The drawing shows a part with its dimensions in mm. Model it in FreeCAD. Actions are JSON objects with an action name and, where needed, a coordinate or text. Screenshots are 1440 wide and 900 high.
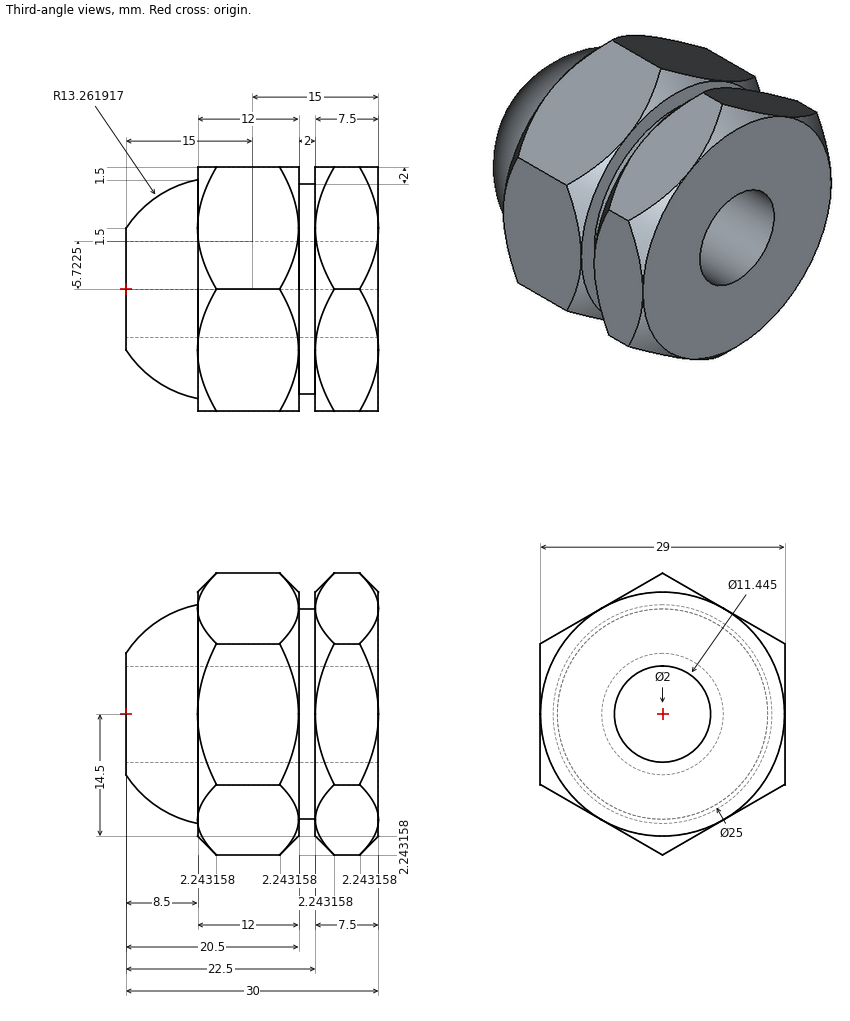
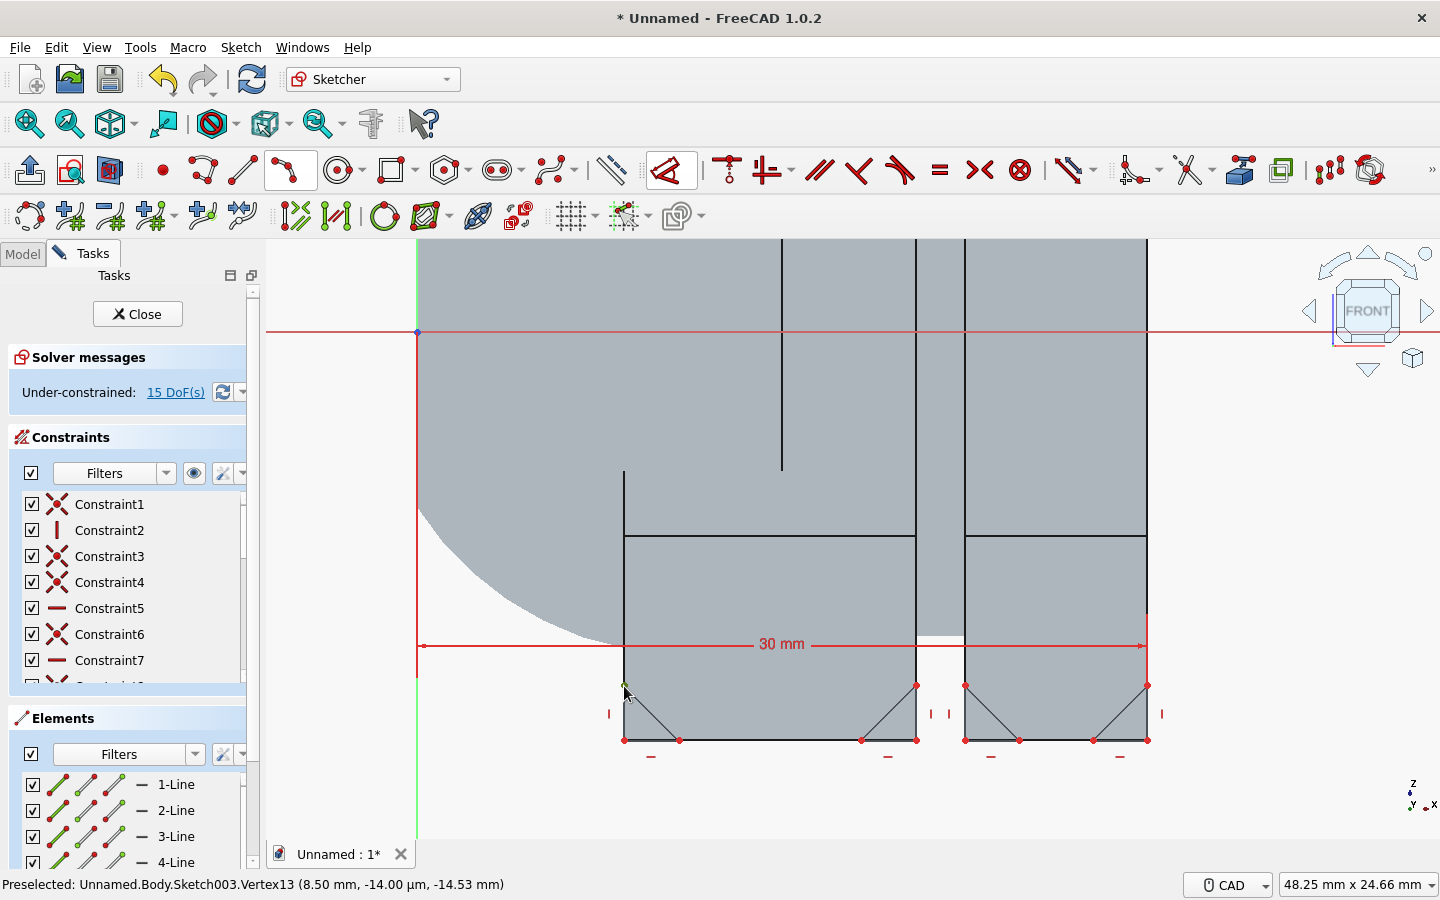
{"action": "left_click", "coordinate": [692, 170]}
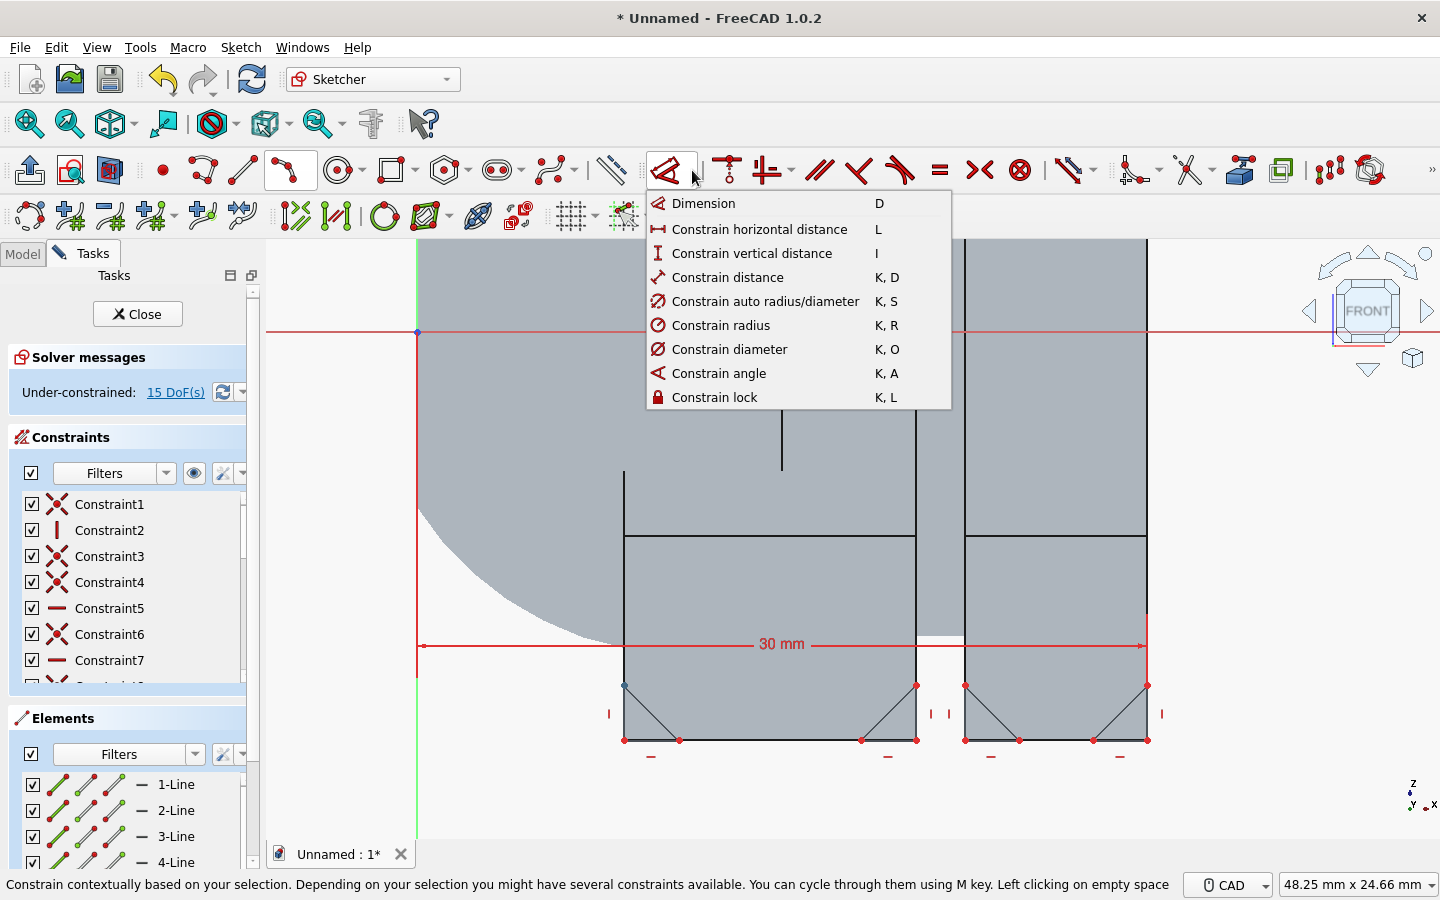
{"action": "left_click", "coordinate": [799, 229]}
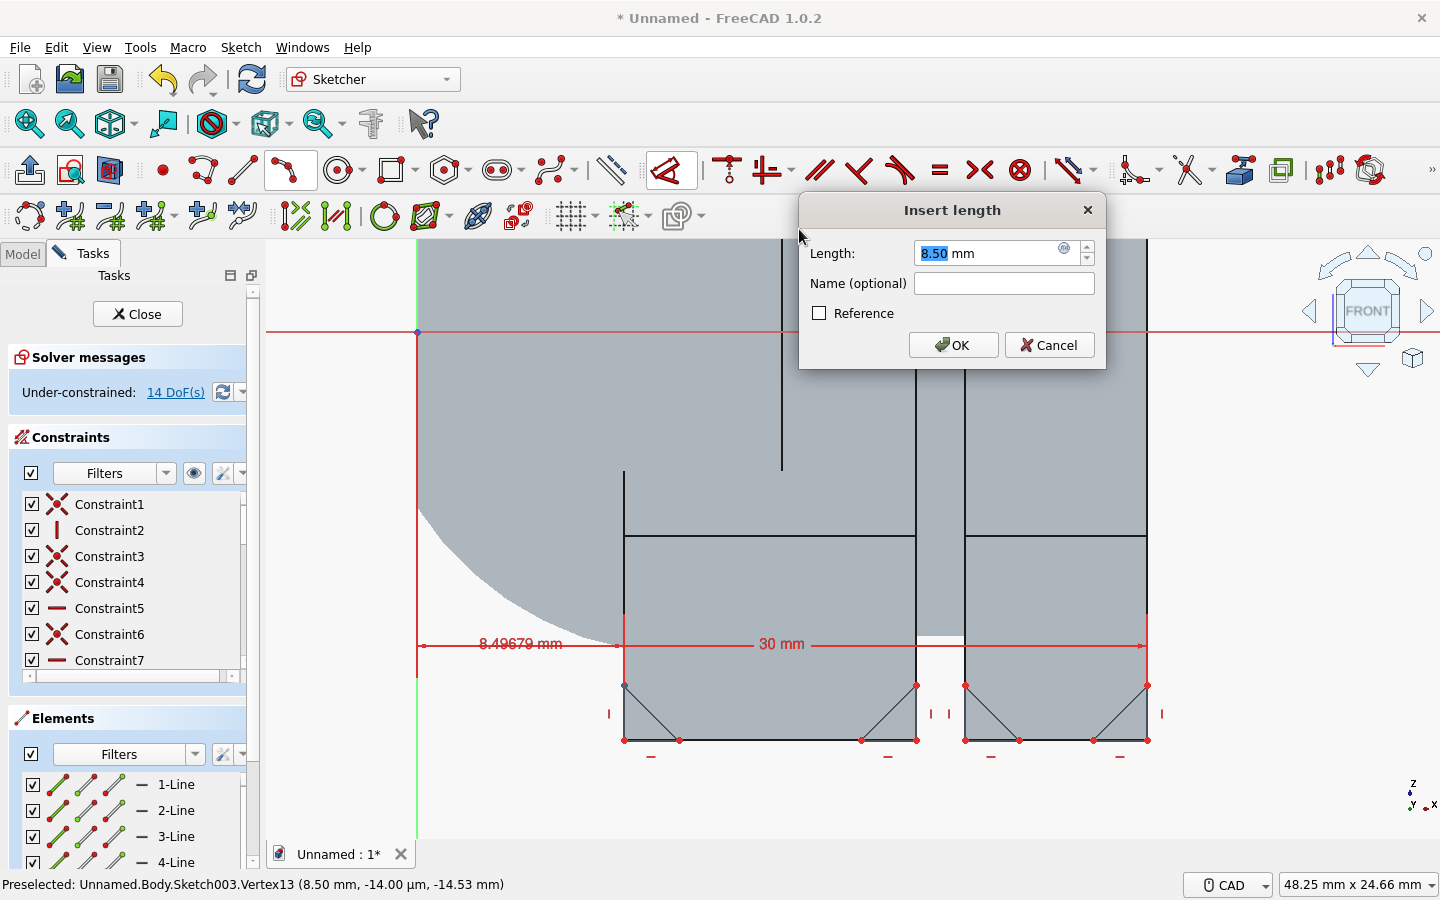
{"action": "type", "text": "8.5"}
{"action": "key", "text": "Return"}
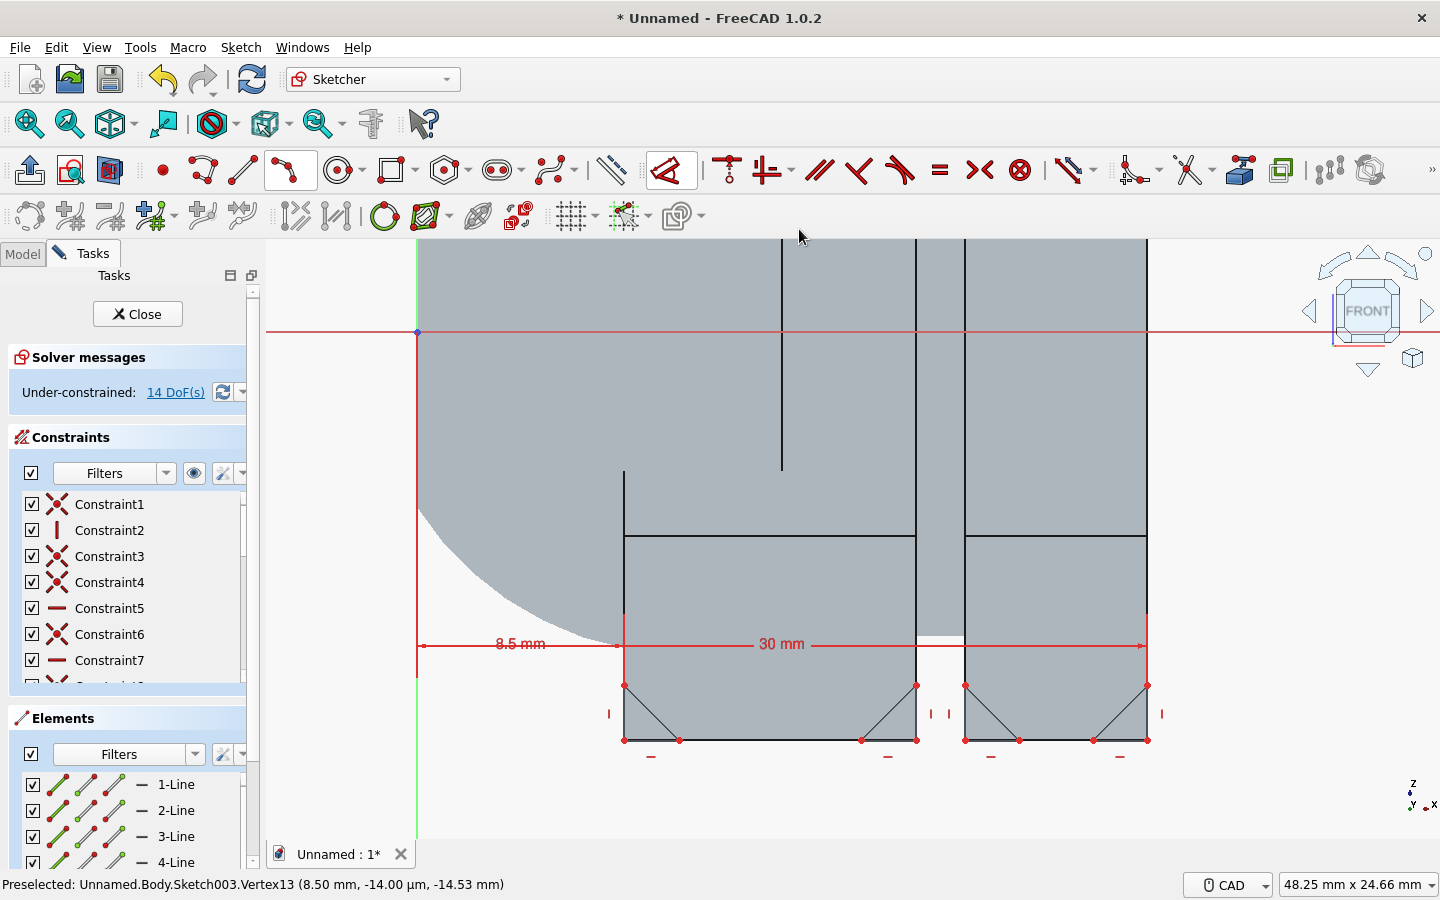
{"action": "left_click", "coordinate": [916, 686]}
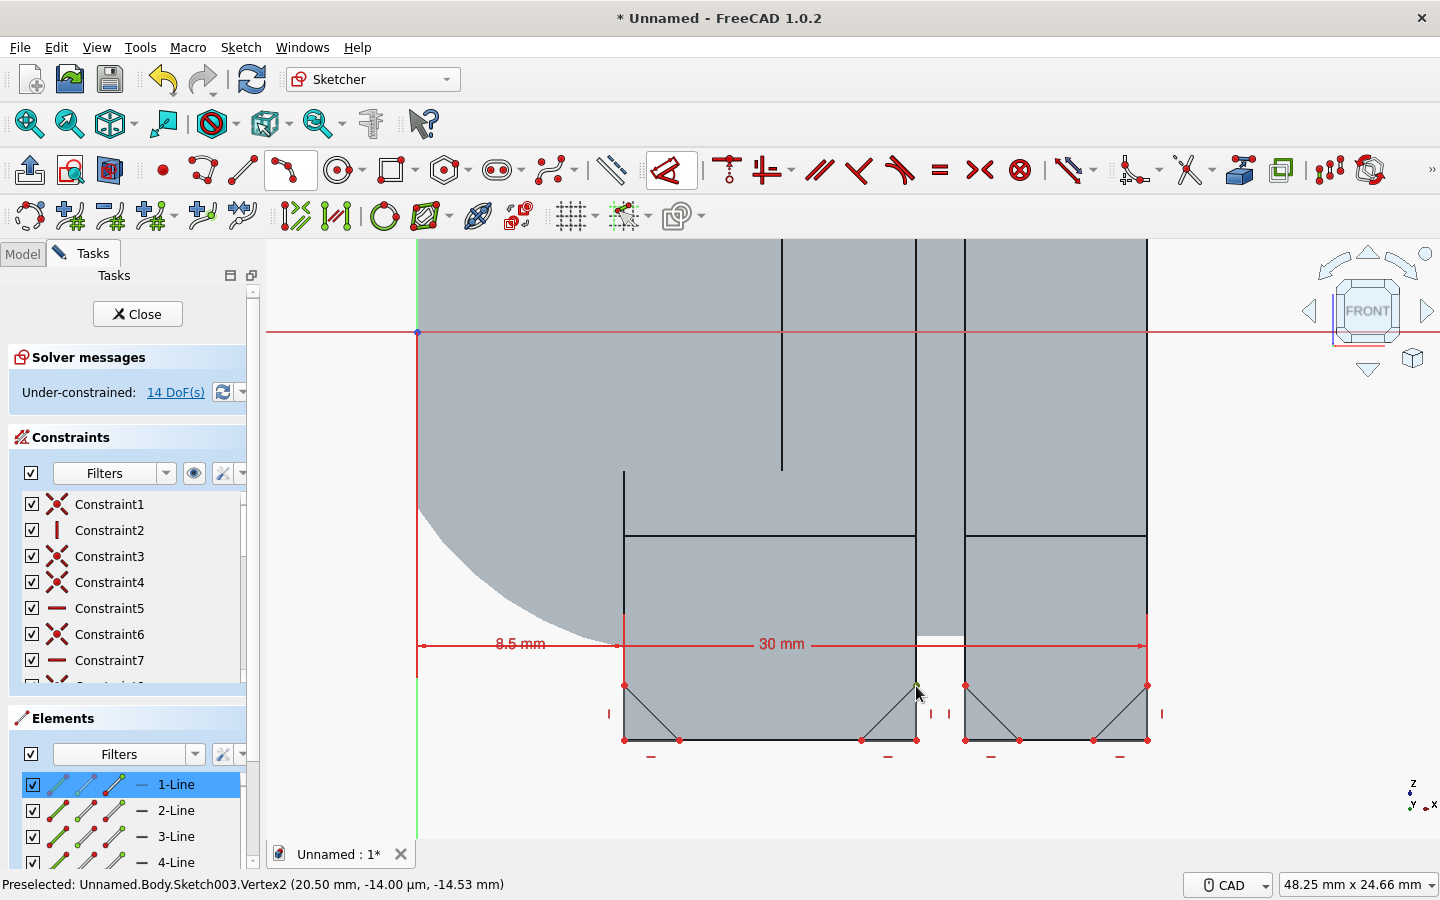
{"action": "left_click", "coordinate": [692, 170]}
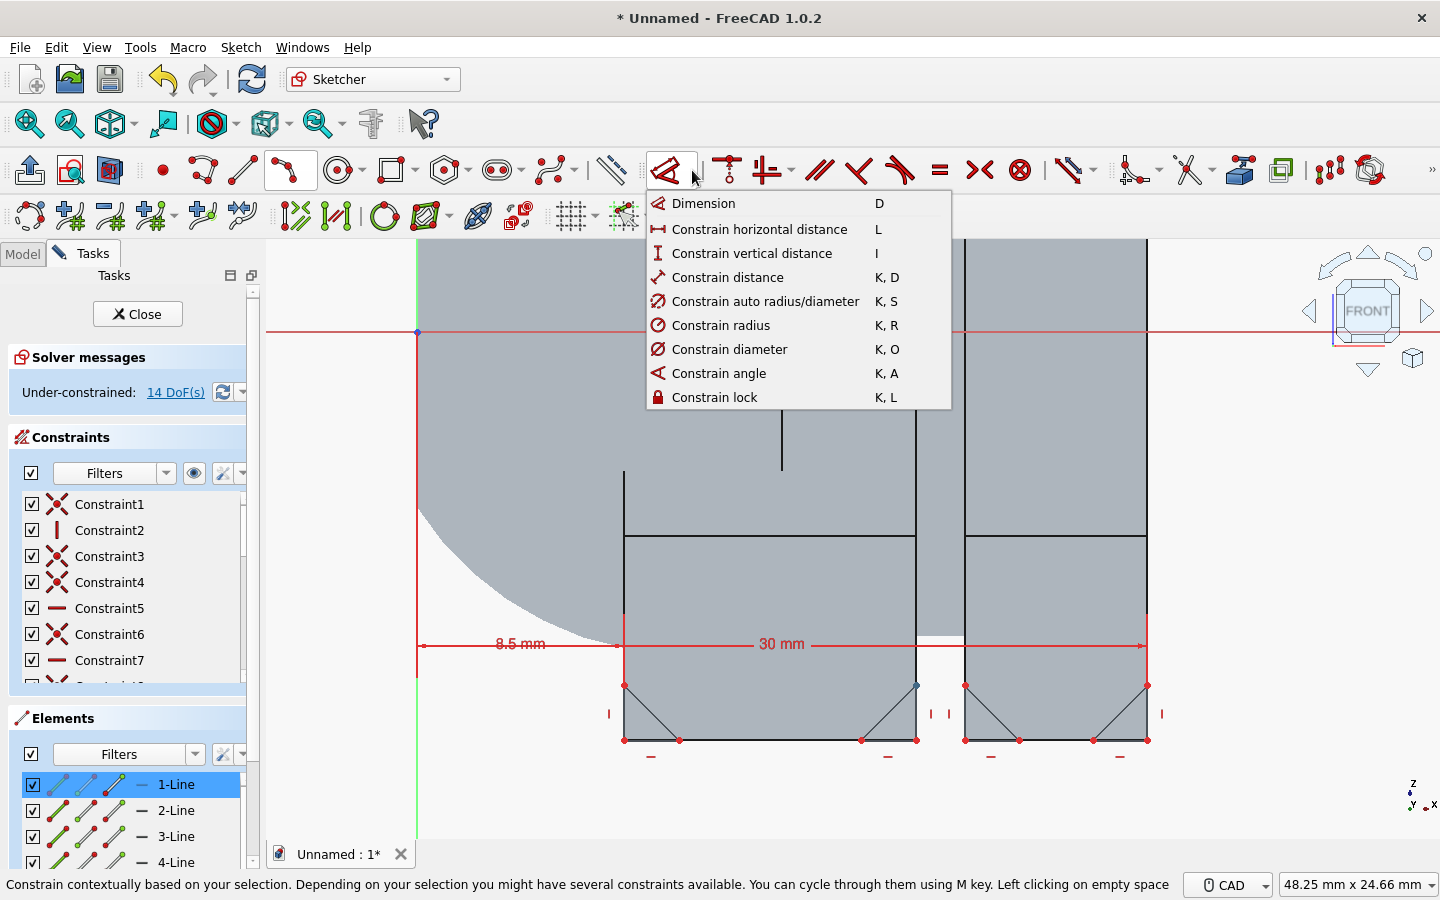
{"action": "left_click", "coordinate": [799, 229]}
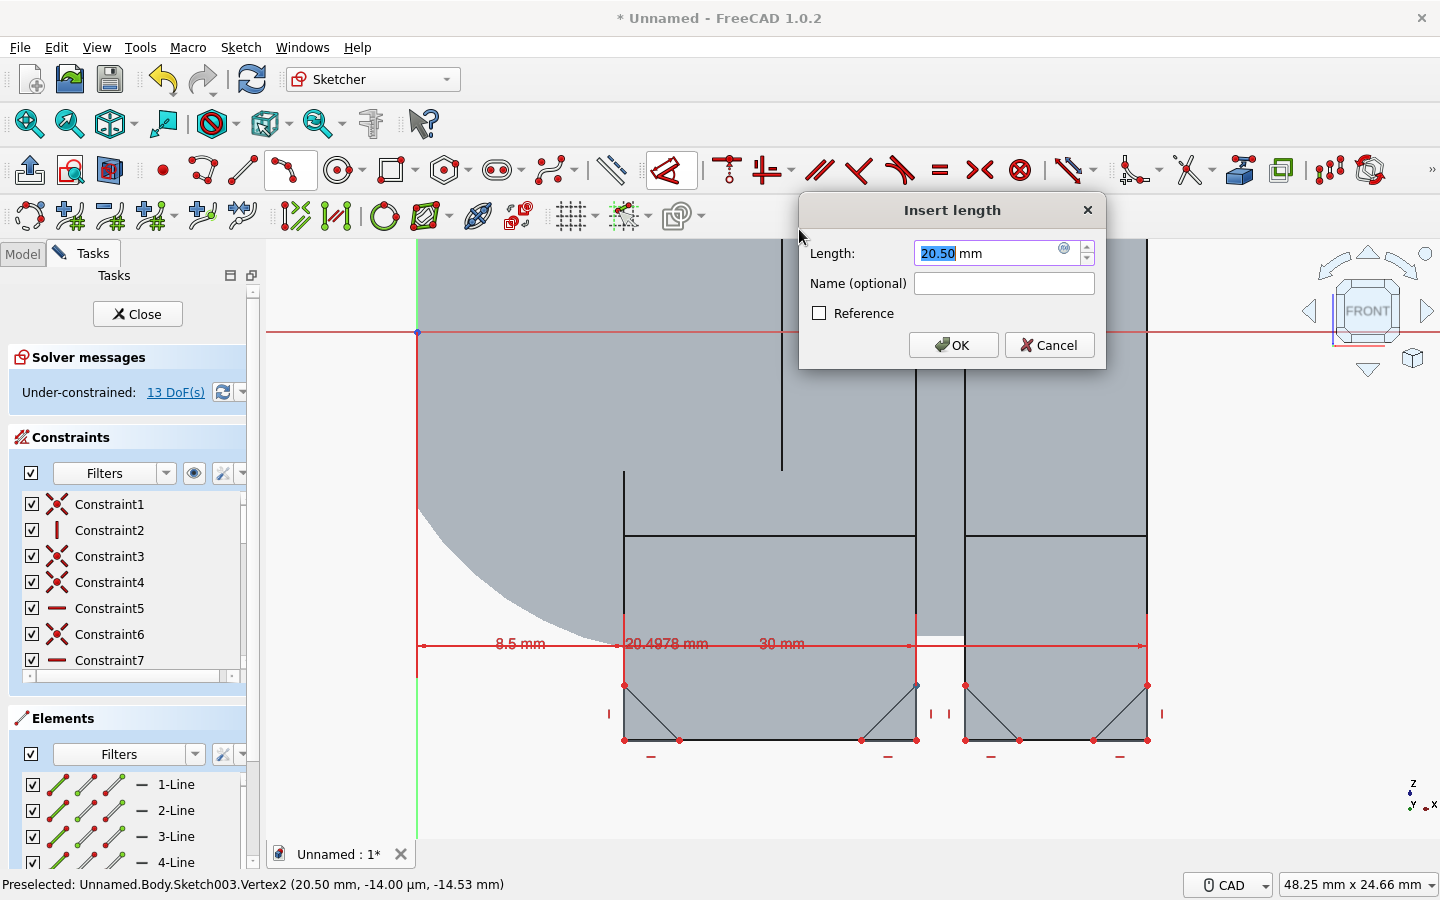
{"action": "type", "text": "20.5"}
{"action": "key", "text": "Return"}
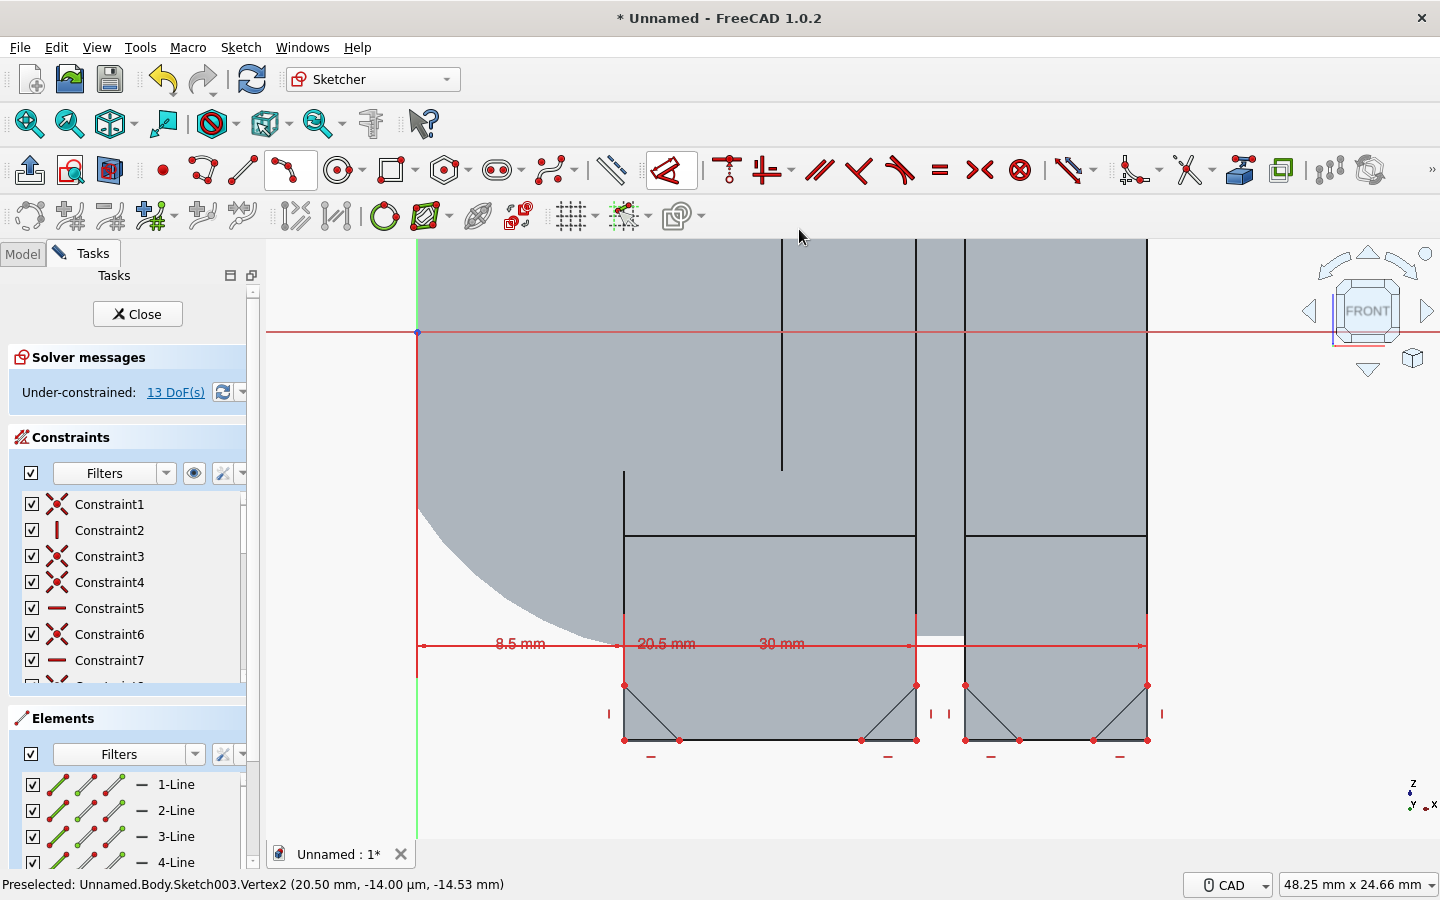
{"action": "left_click", "coordinate": [916, 686]}